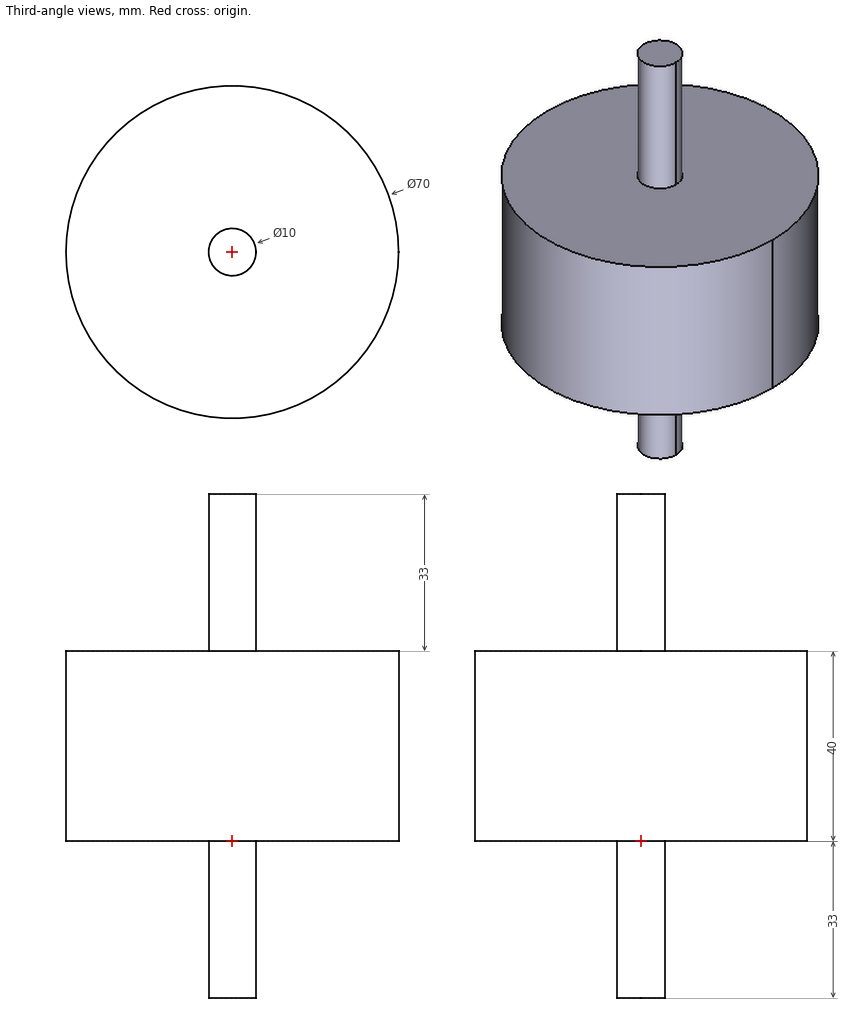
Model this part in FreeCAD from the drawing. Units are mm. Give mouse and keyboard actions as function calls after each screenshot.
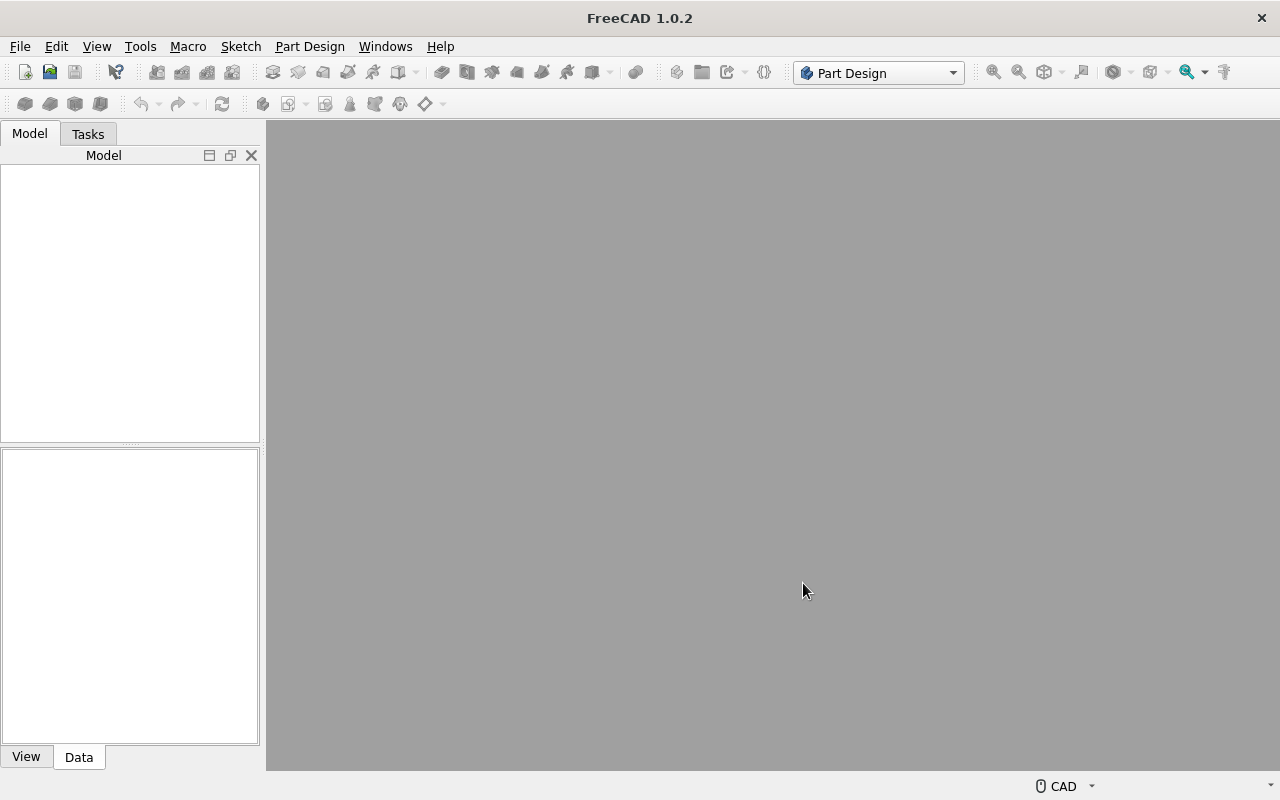
key(ctrl+n)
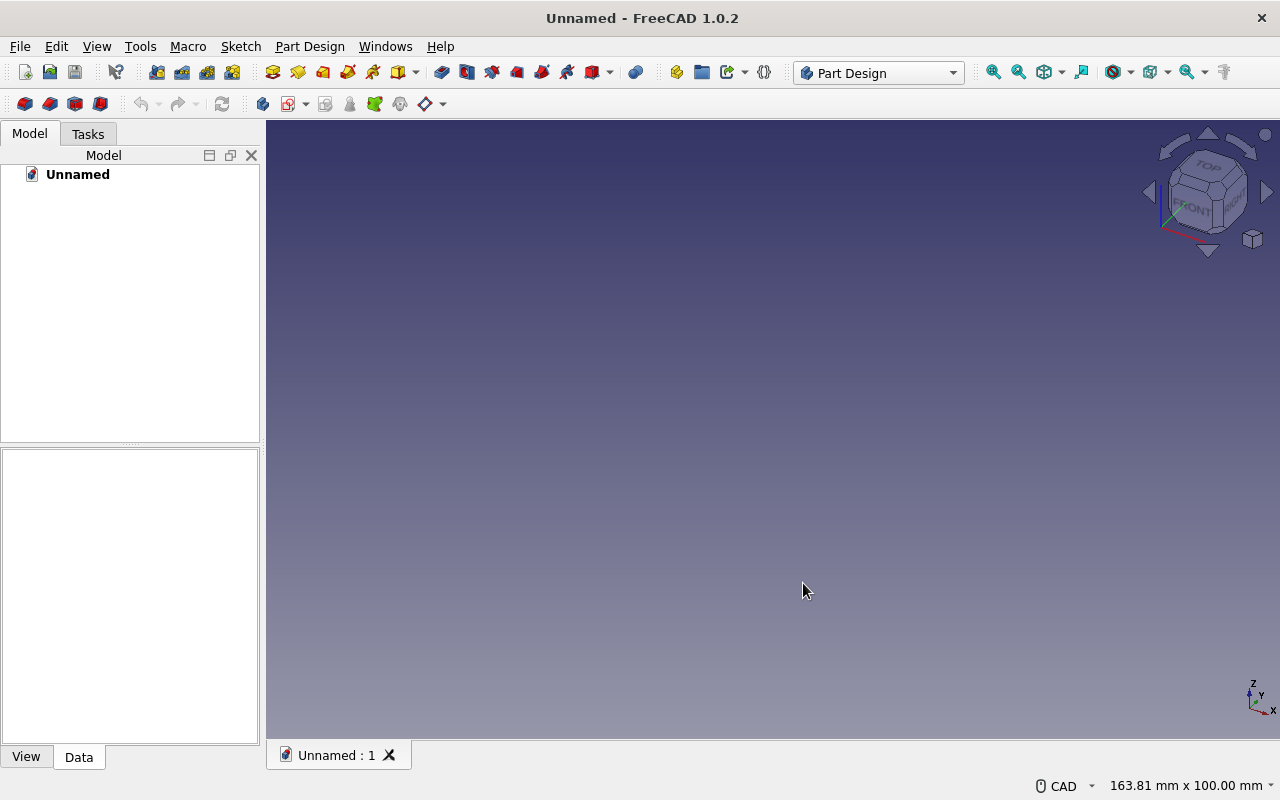
click(288, 104)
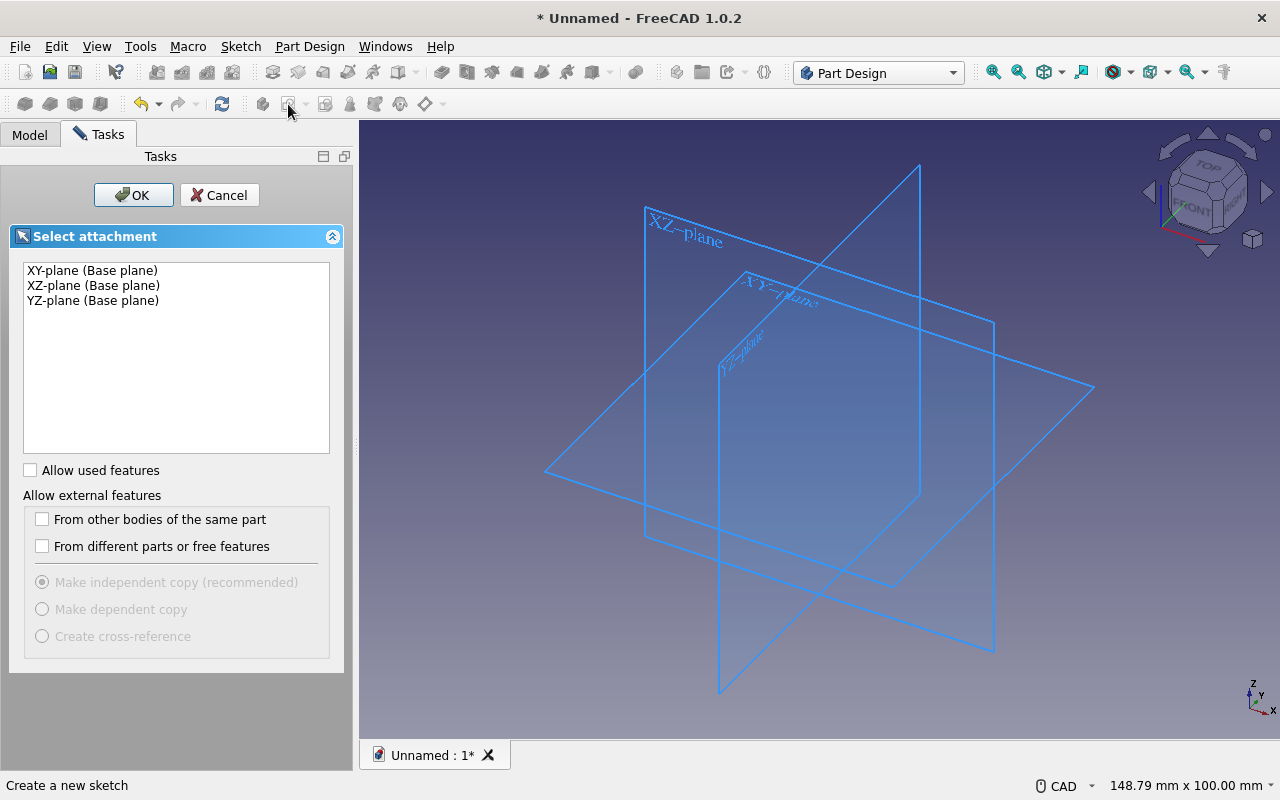
click(84, 270)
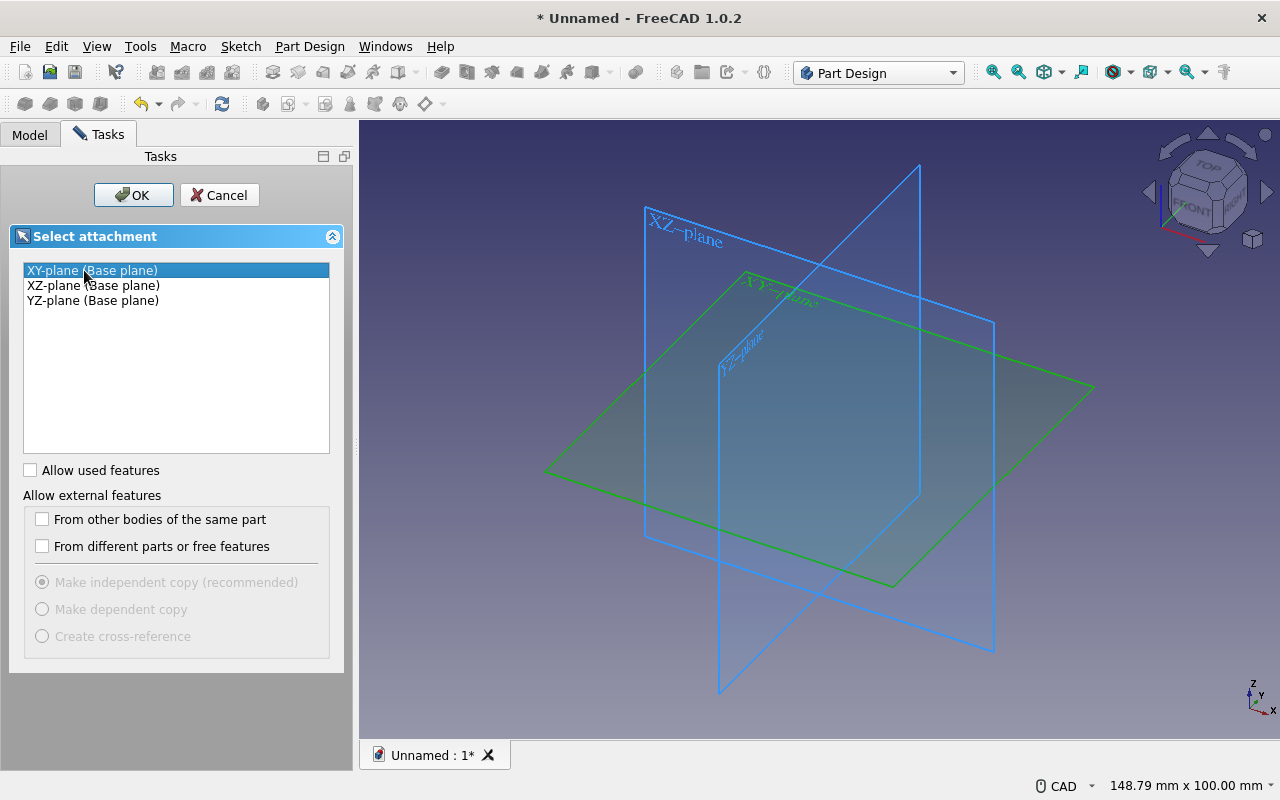
click(134, 195)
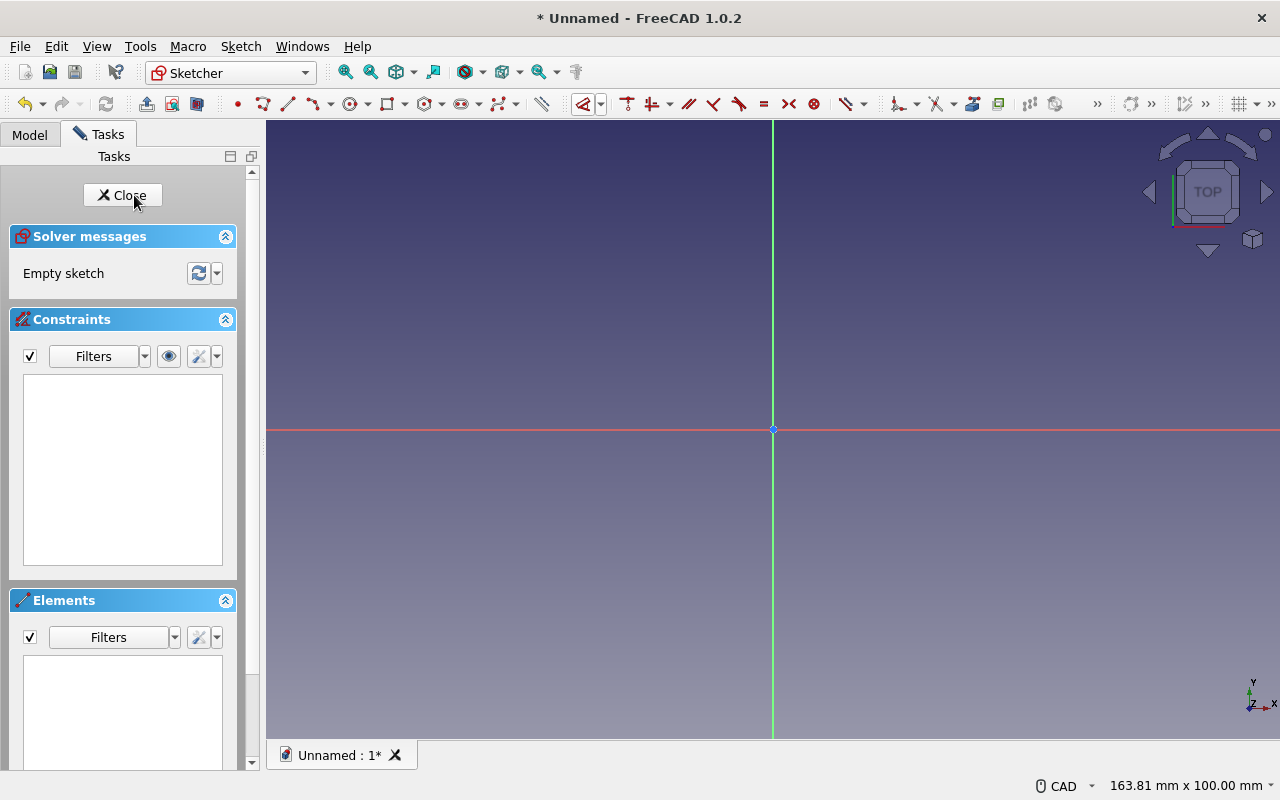
click(350, 104)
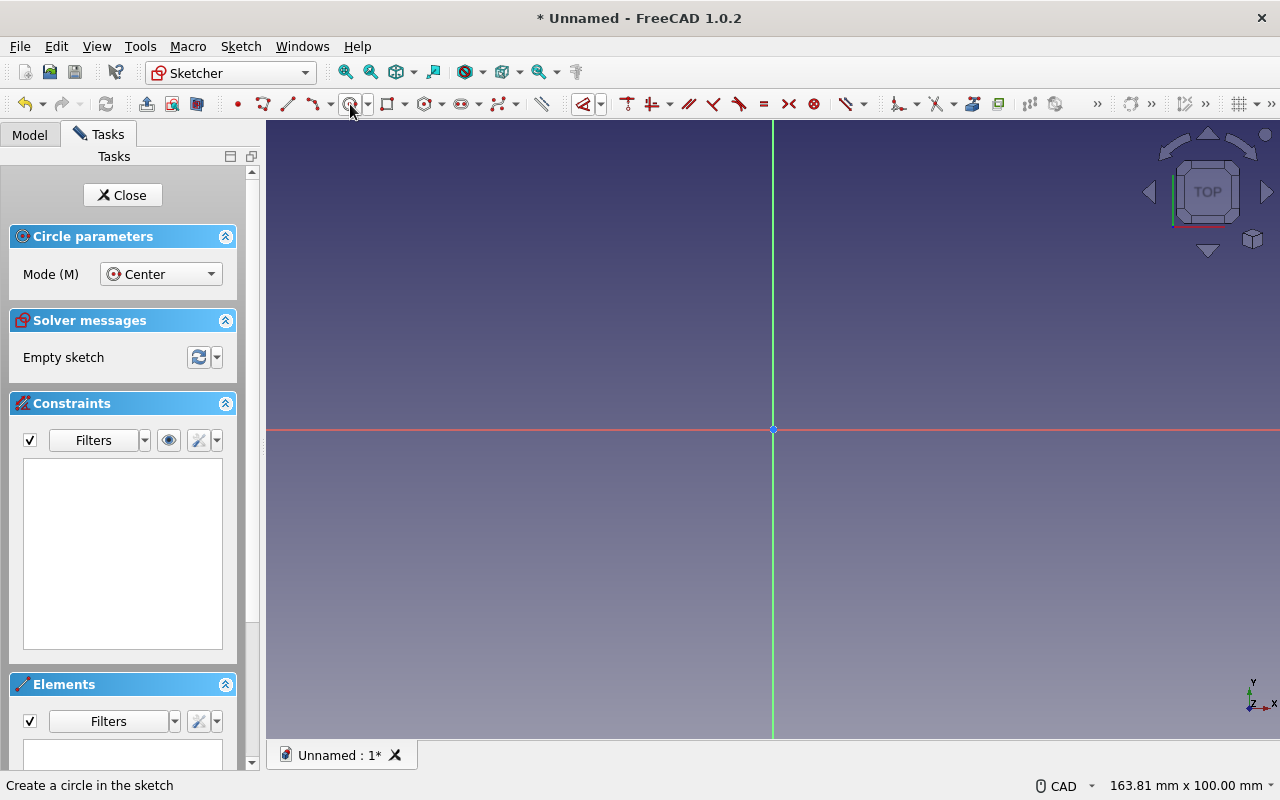
click(773, 430)
click(926, 276)
key(Escape)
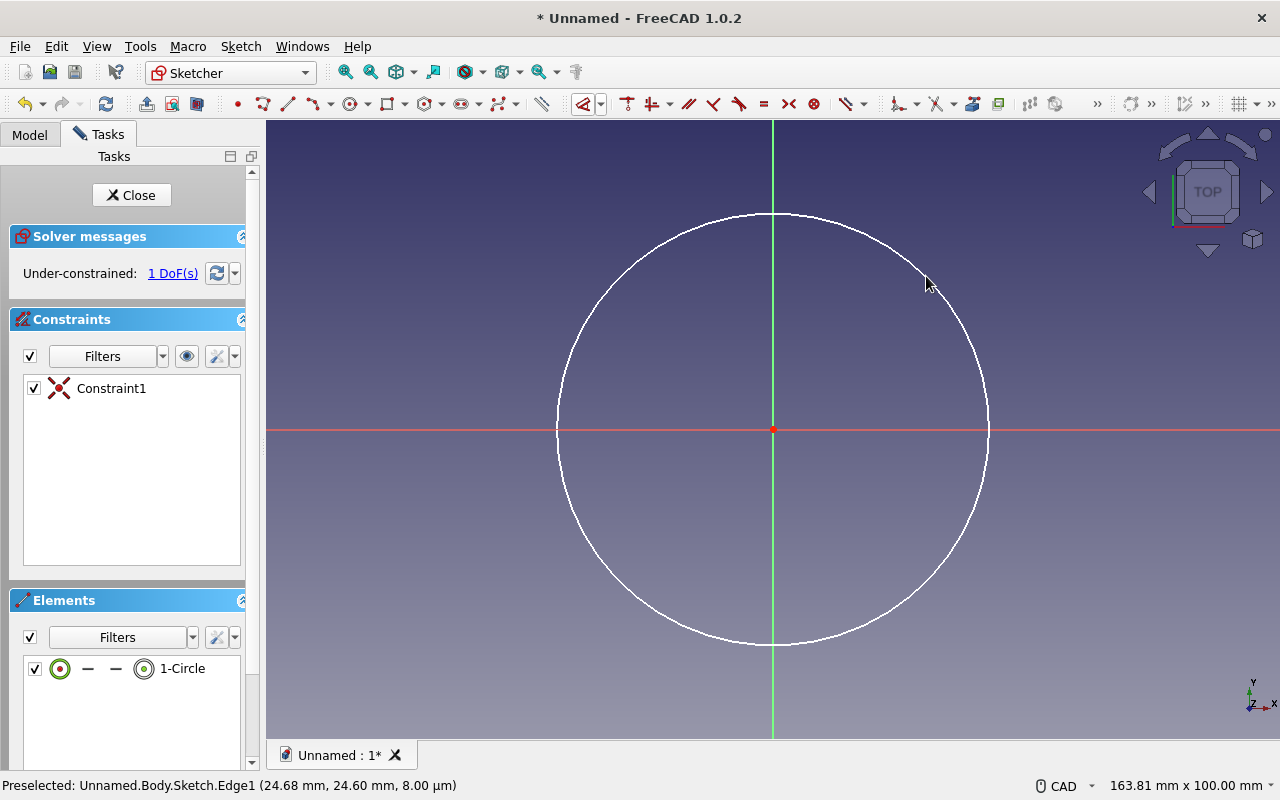
key(d)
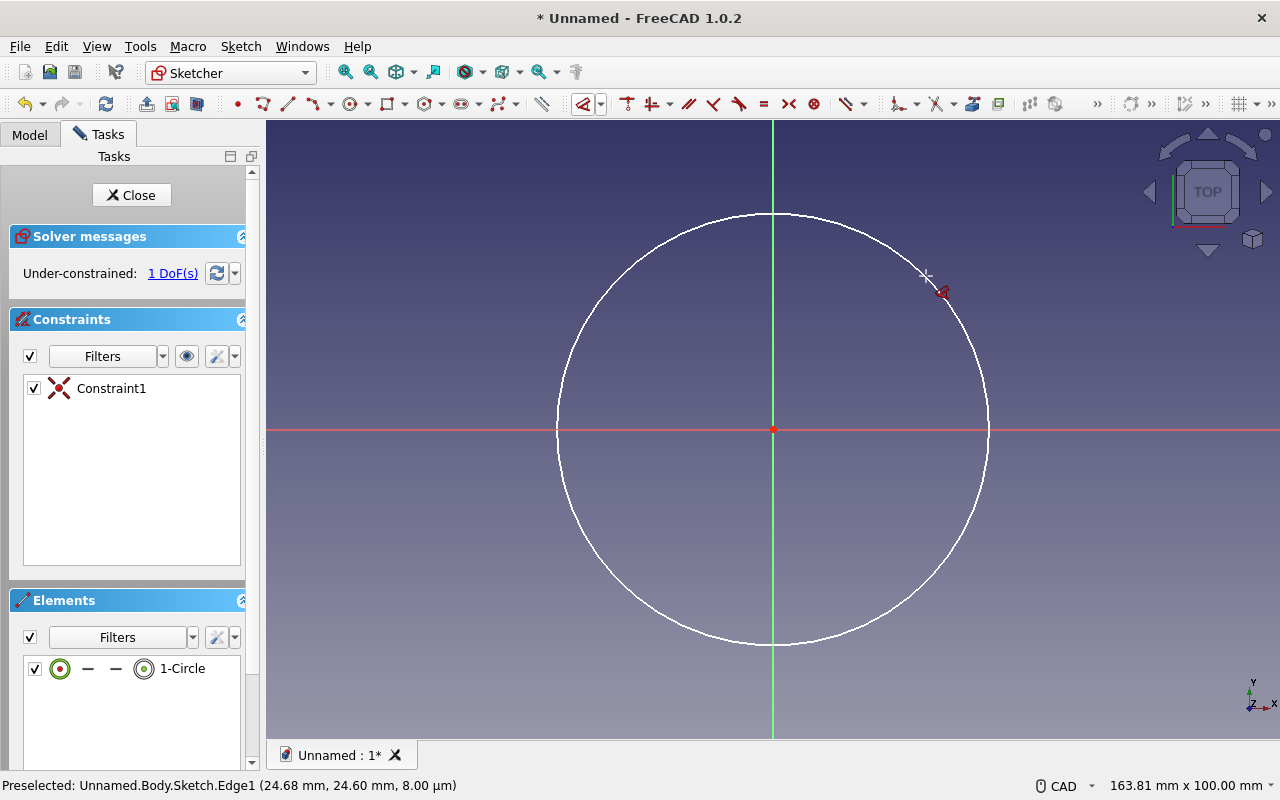
click(925, 276)
click(948, 253)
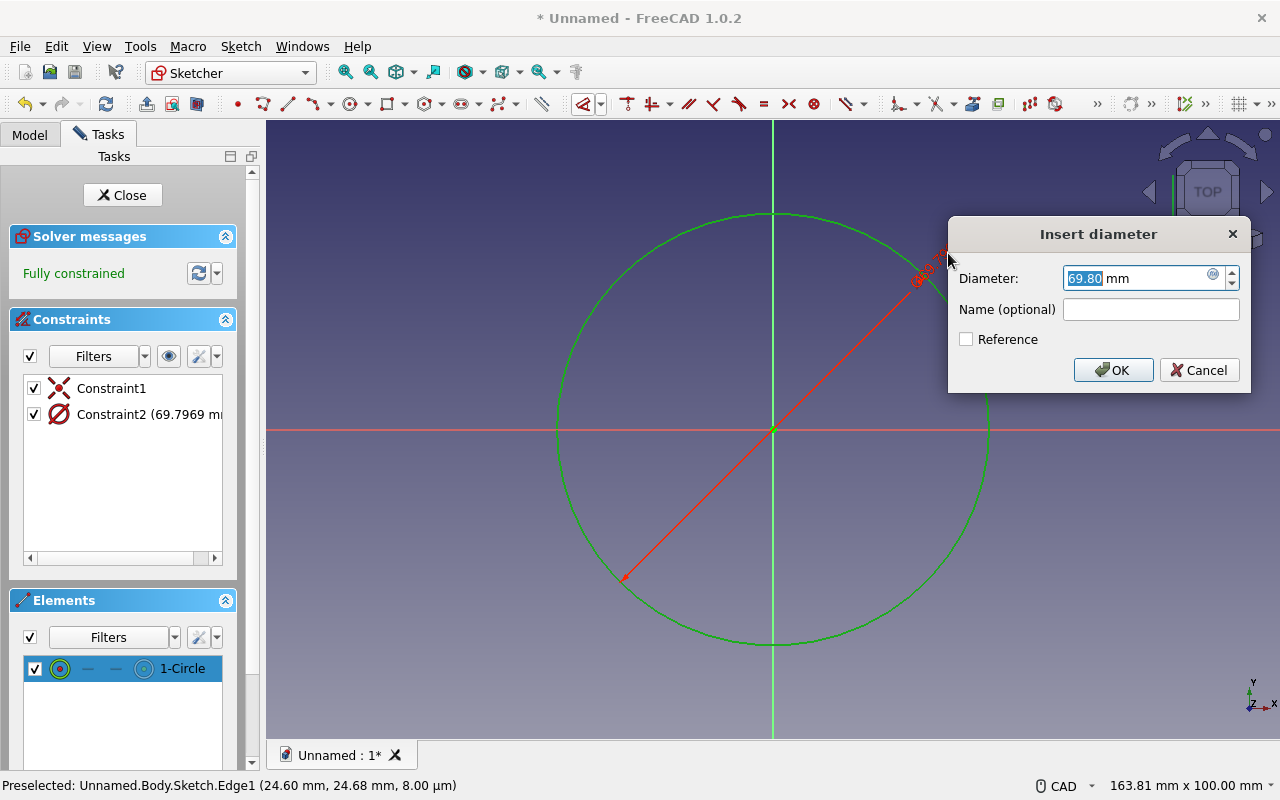
text(70)
key(Return)
key(Escape)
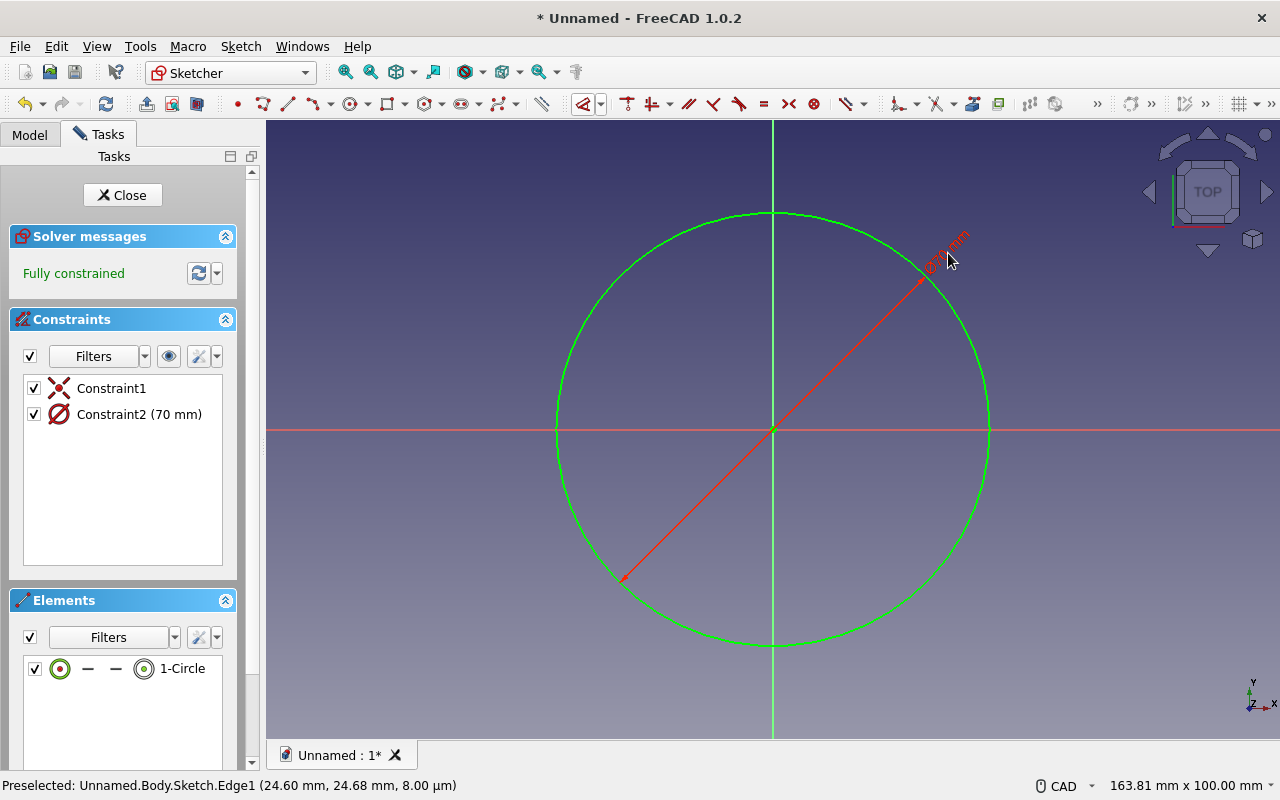
click(123, 195)